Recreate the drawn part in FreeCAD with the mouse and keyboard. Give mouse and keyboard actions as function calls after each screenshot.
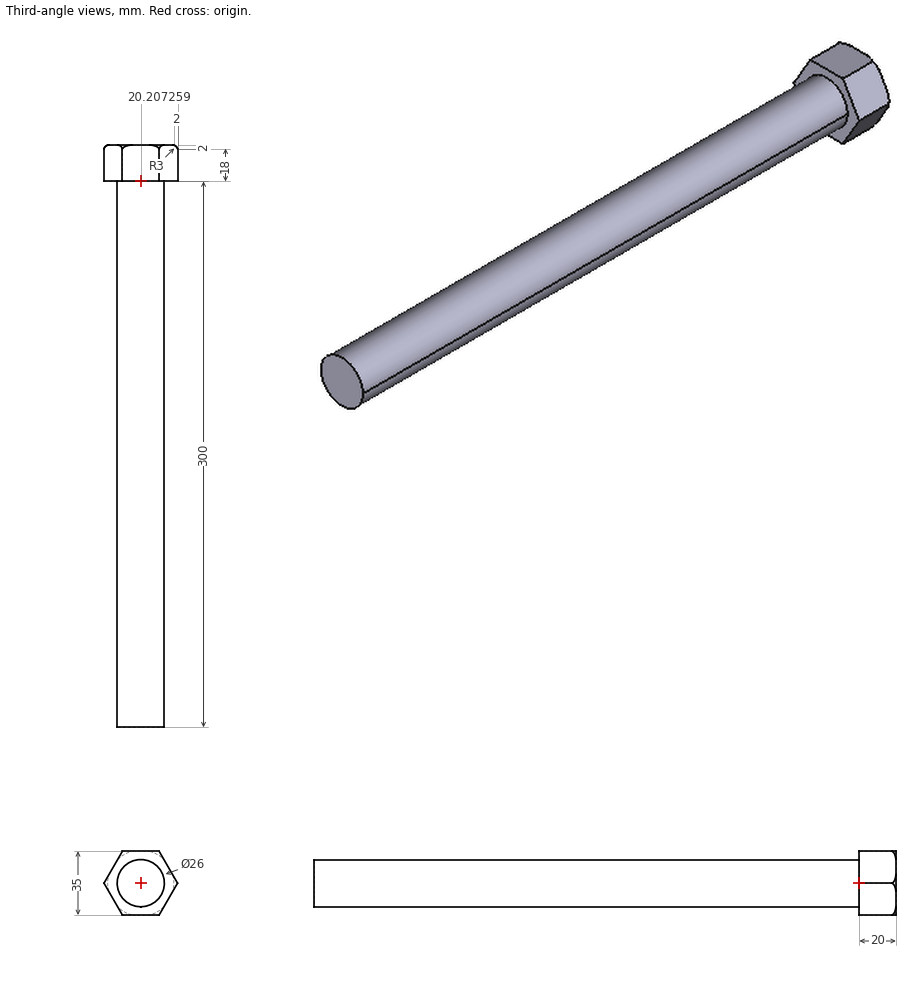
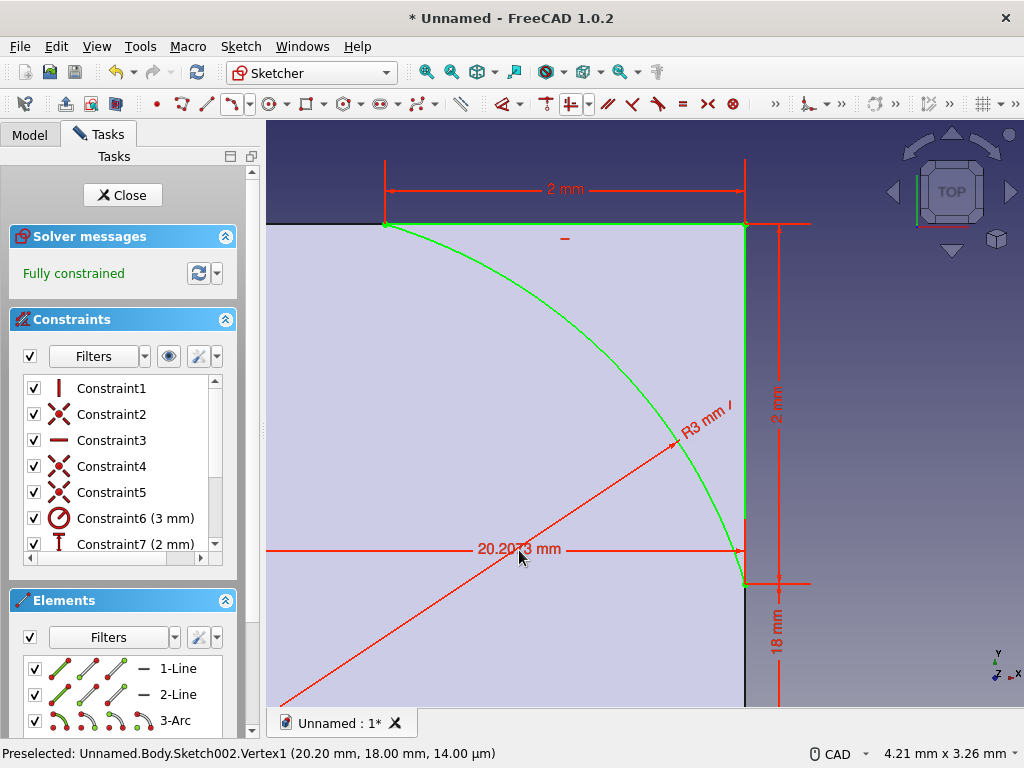
click(123, 195)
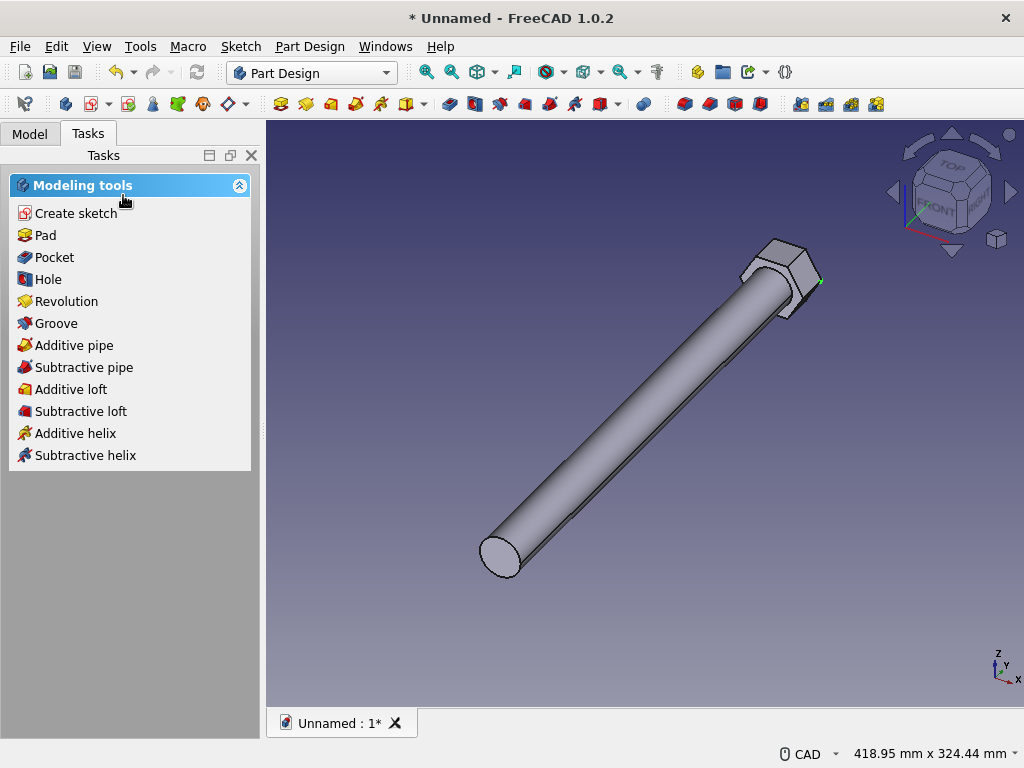
click(500, 104)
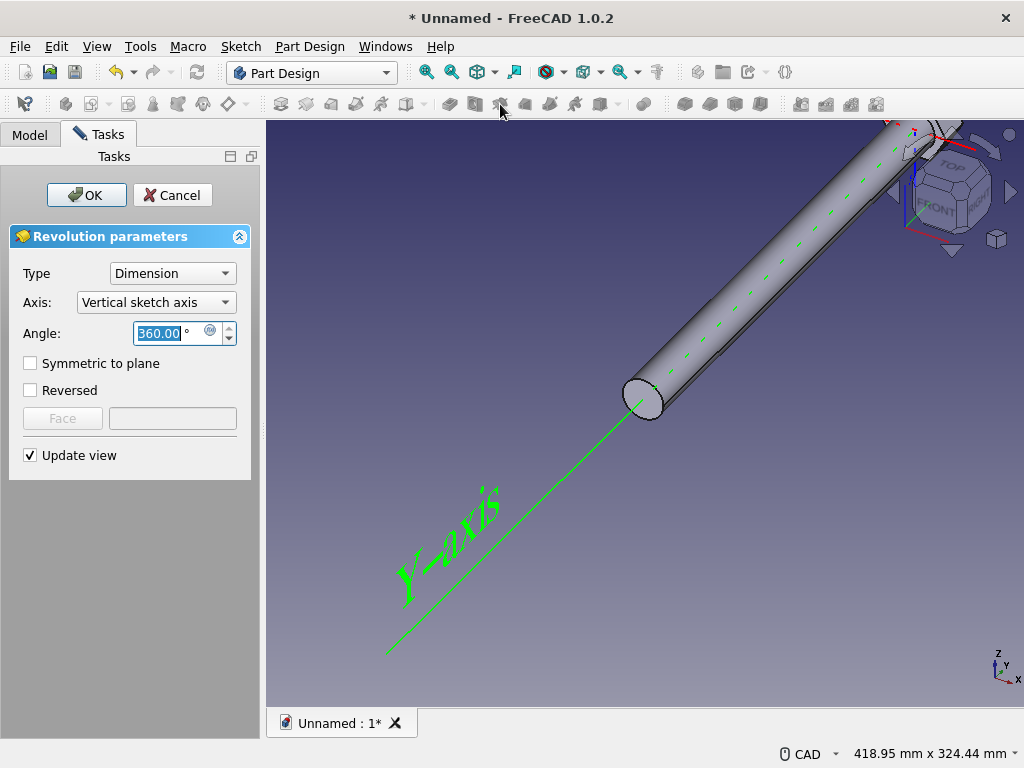
click(87, 195)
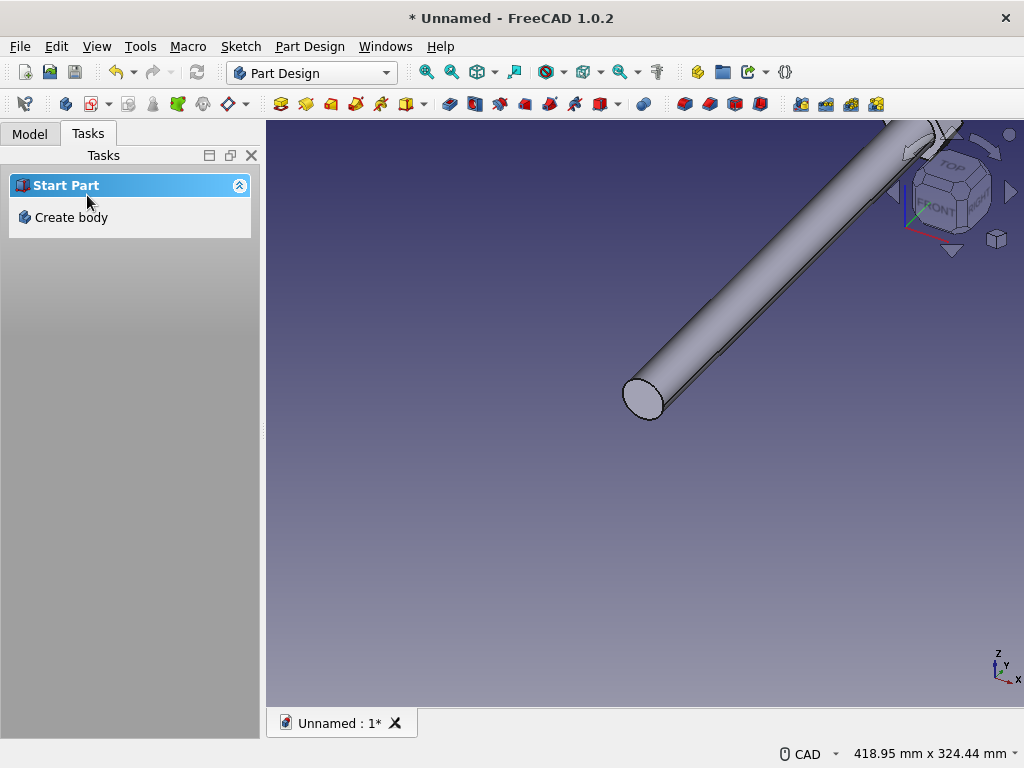
key(0)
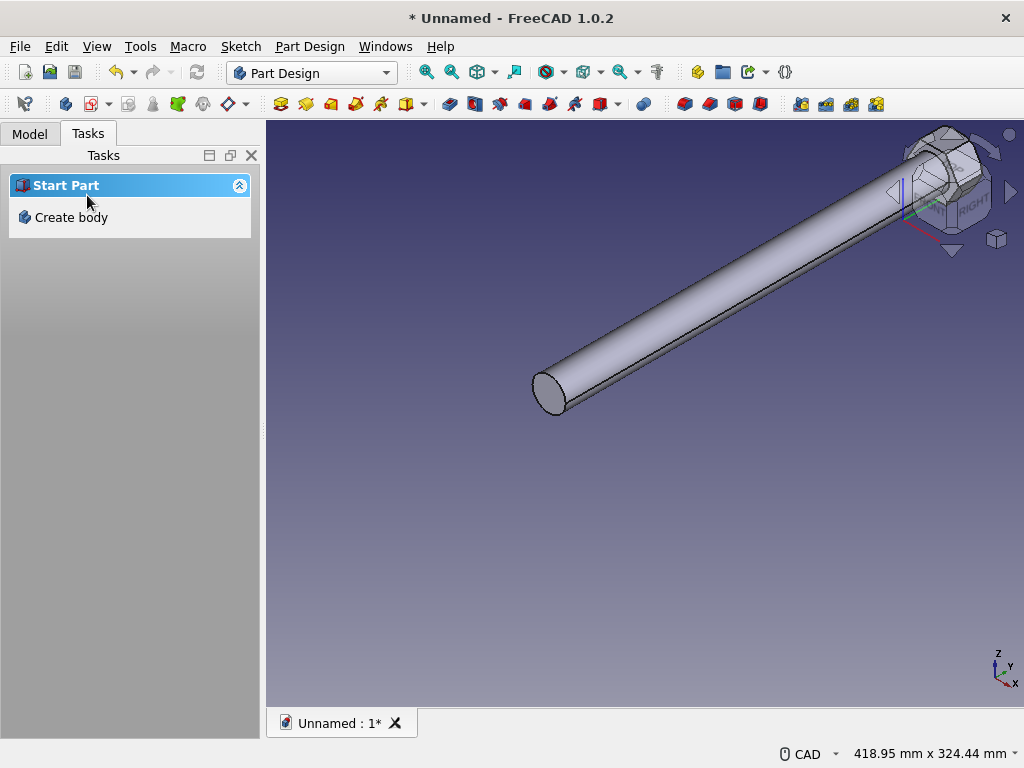
key(v)
key(f)